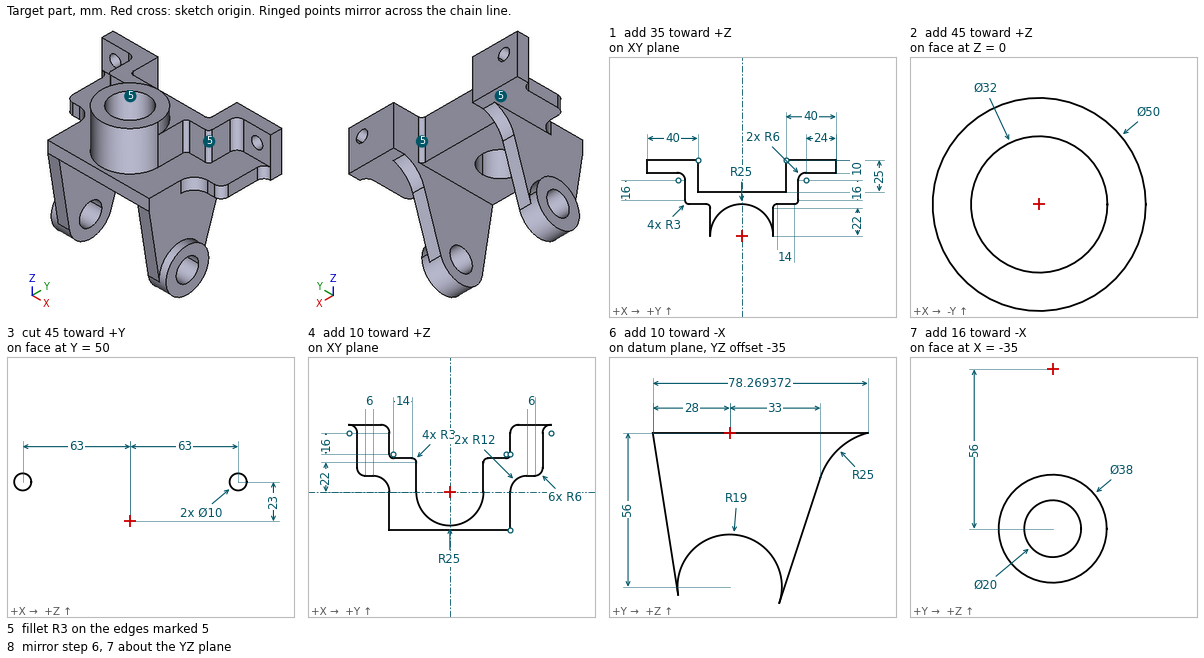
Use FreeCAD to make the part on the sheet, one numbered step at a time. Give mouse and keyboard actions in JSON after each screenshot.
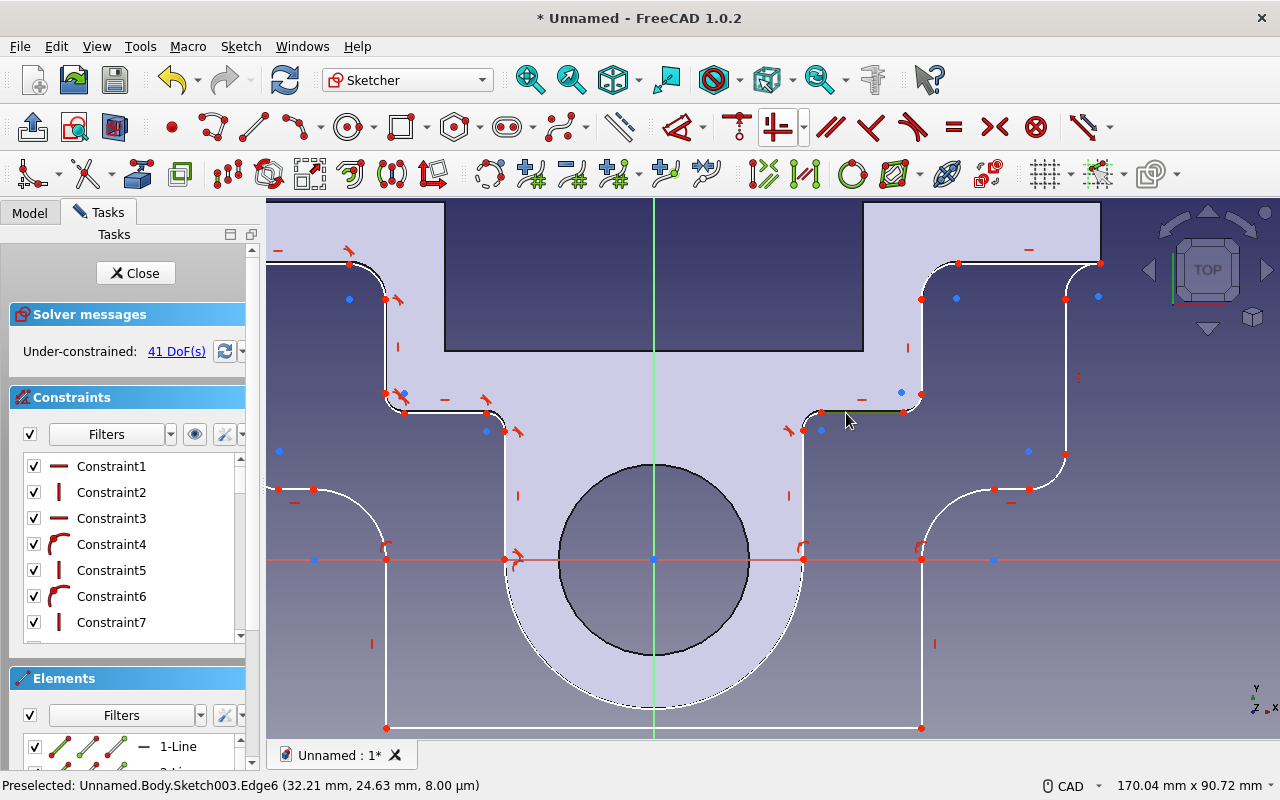
{"action": "left_click", "coordinate": [809, 418]}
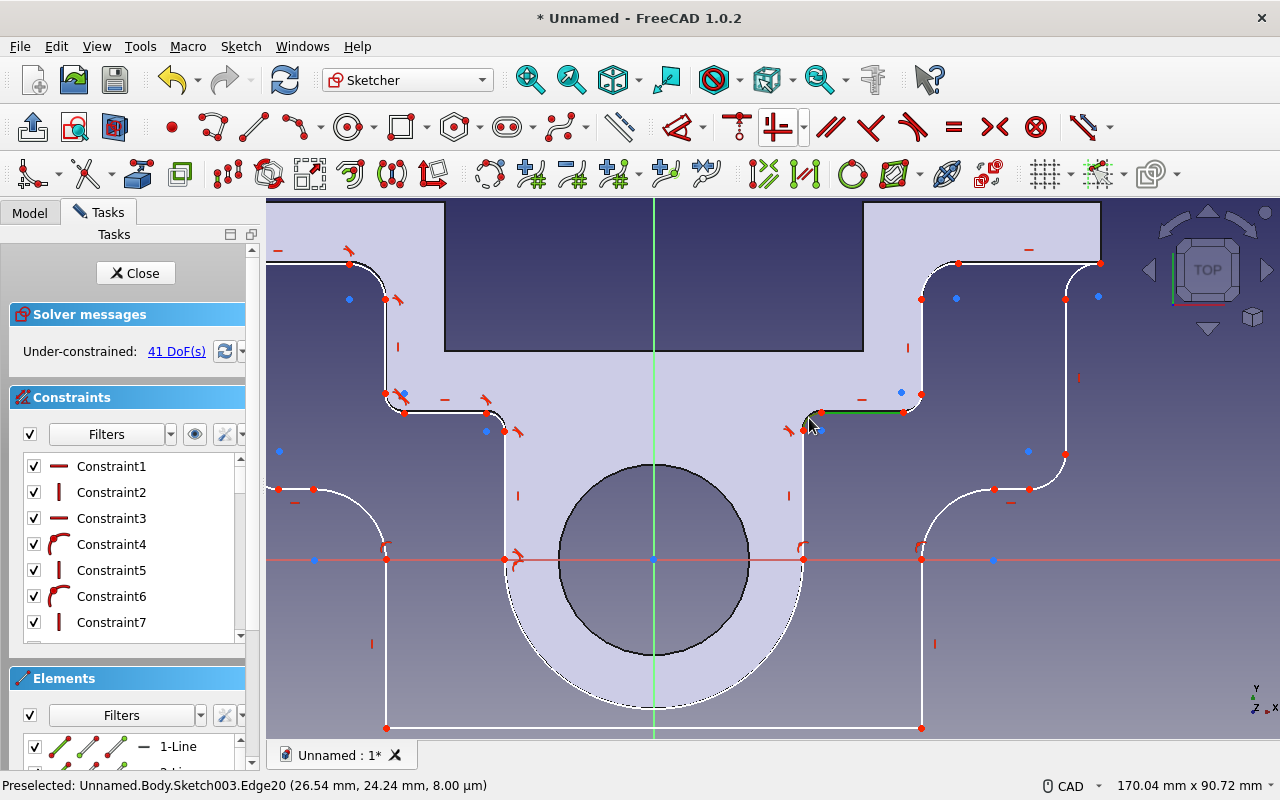
{"action": "left_click", "coordinate": [913, 128]}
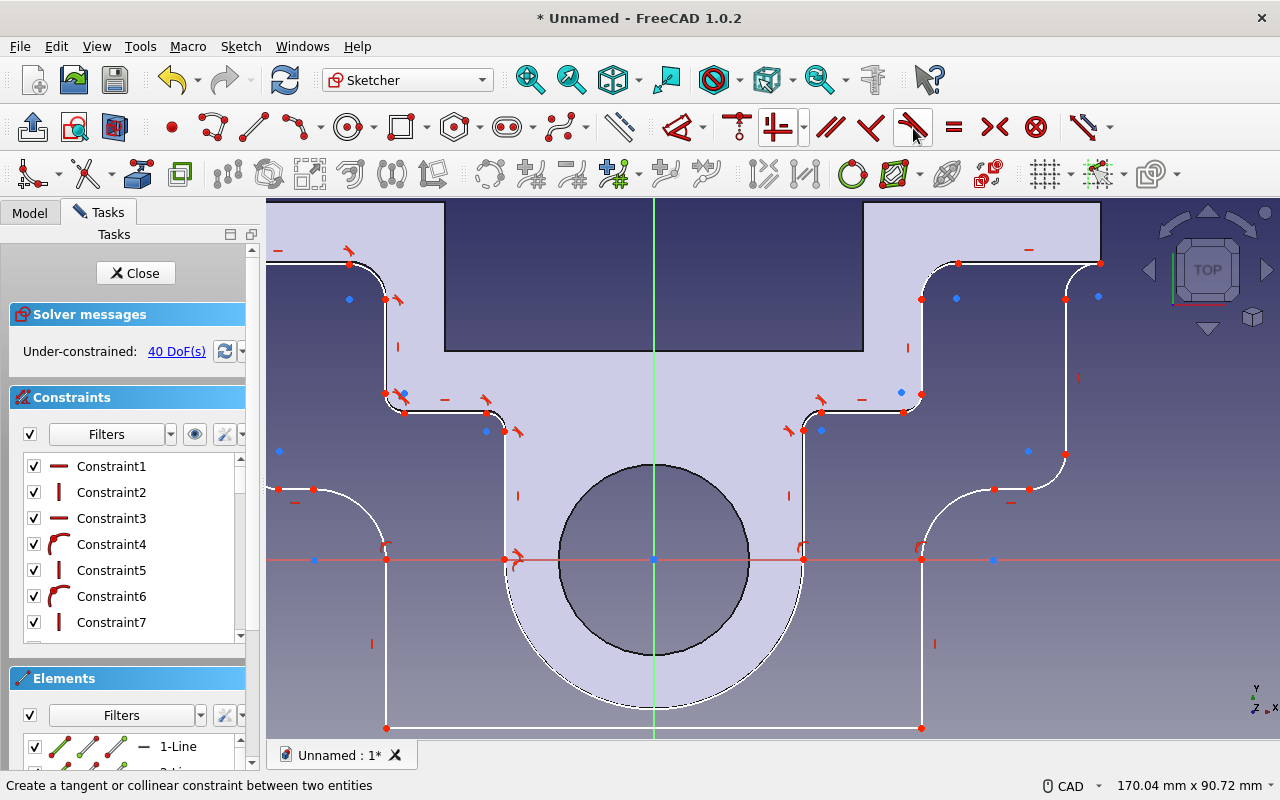
{"action": "left_click", "coordinate": [846, 413]}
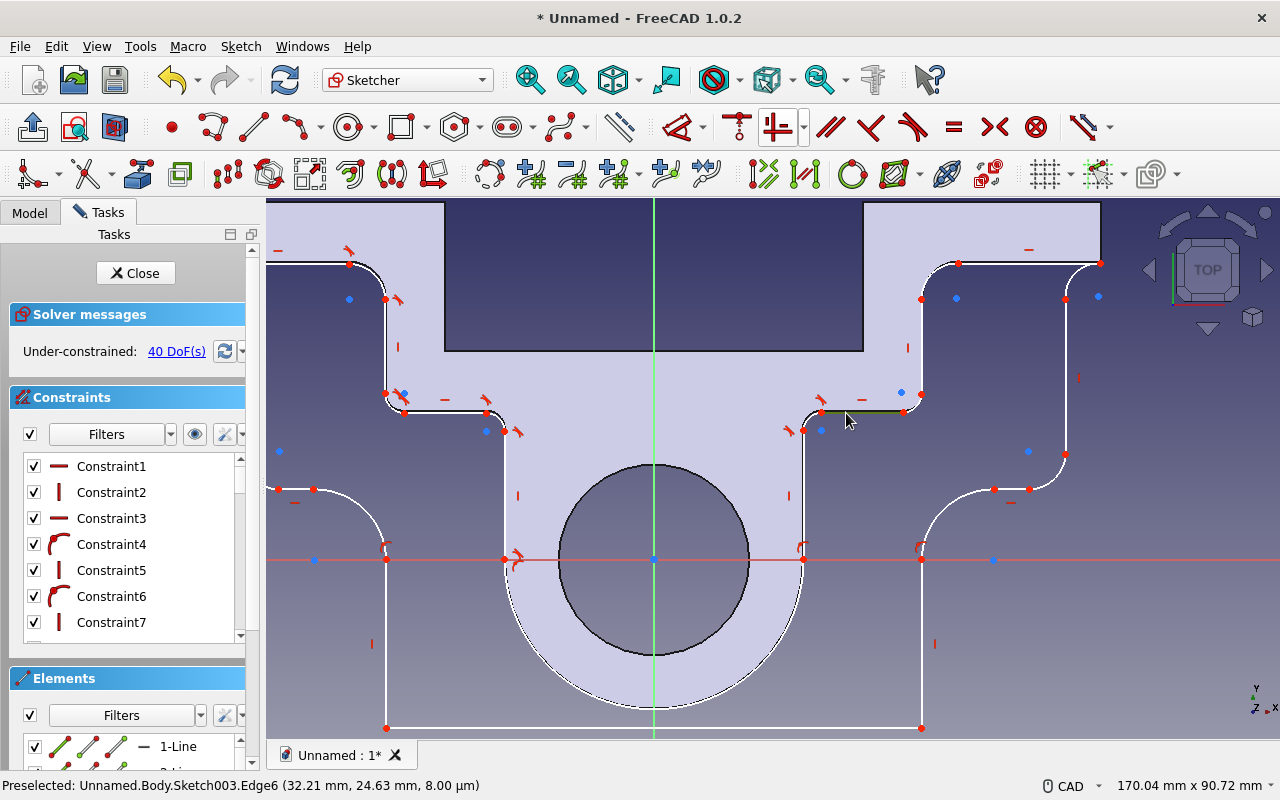
{"action": "left_click", "coordinate": [916, 407]}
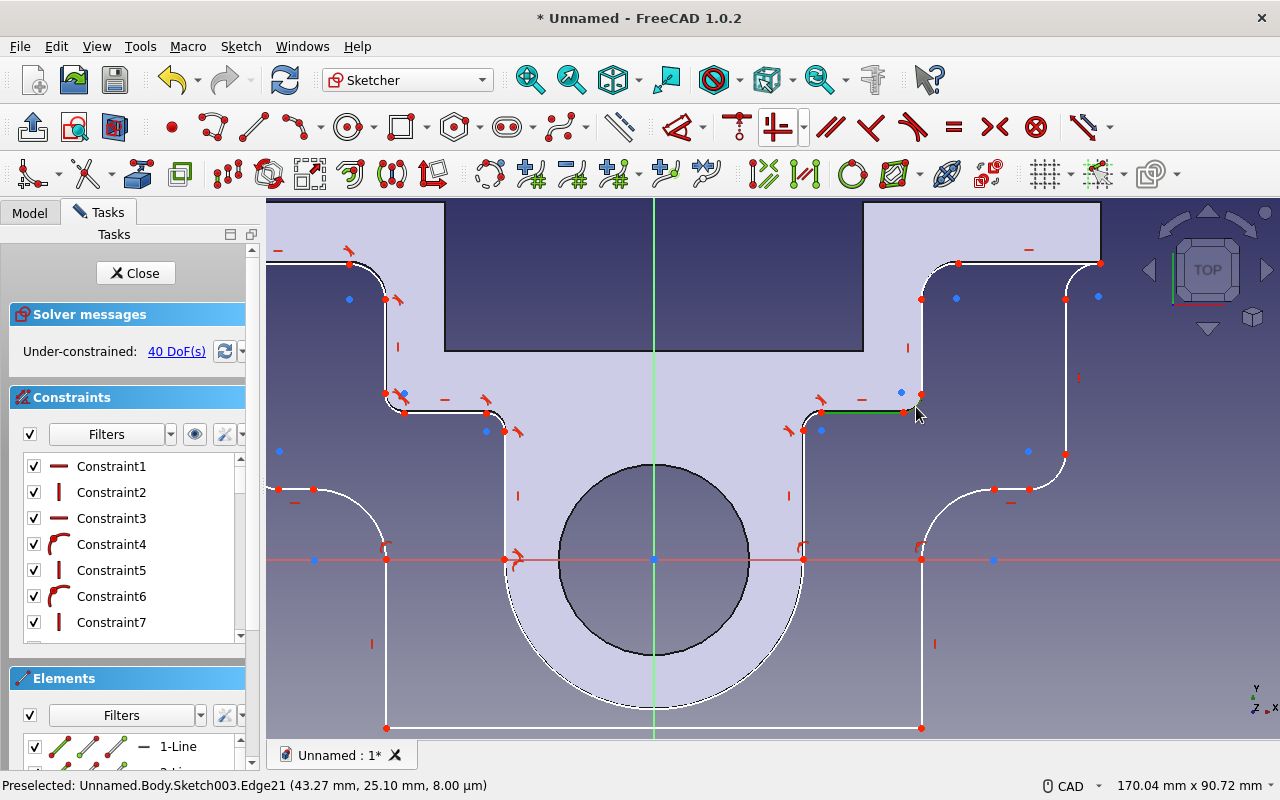
{"action": "left_click", "coordinate": [913, 128]}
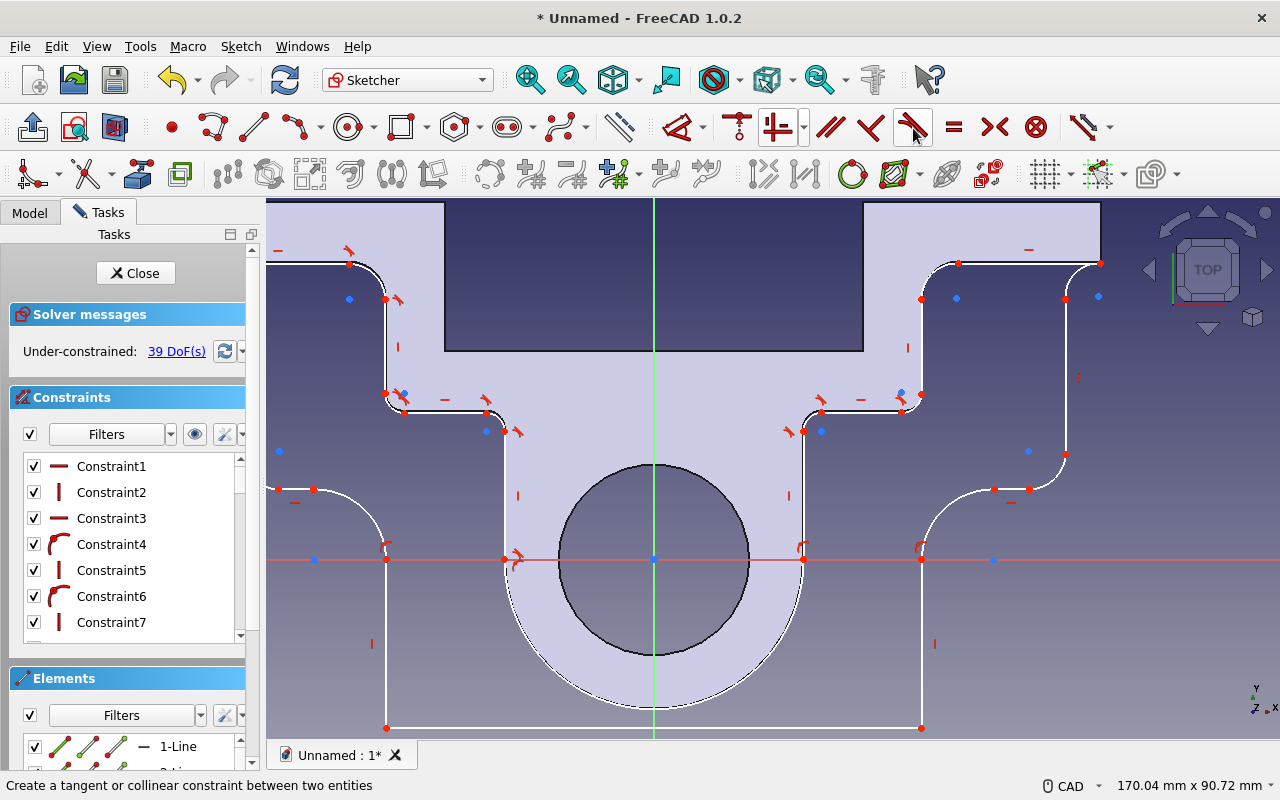
{"action": "left_click", "coordinate": [922, 366]}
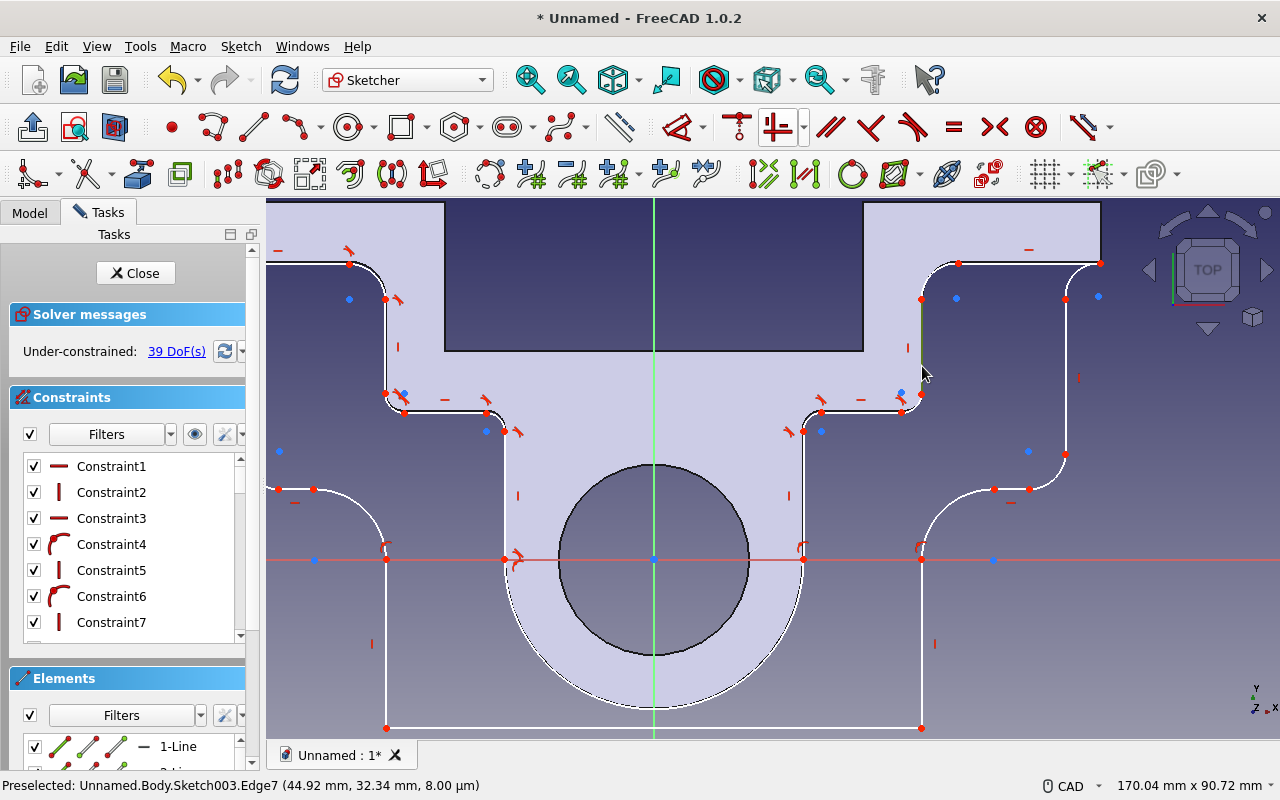
{"action": "left_click", "coordinate": [915, 408]}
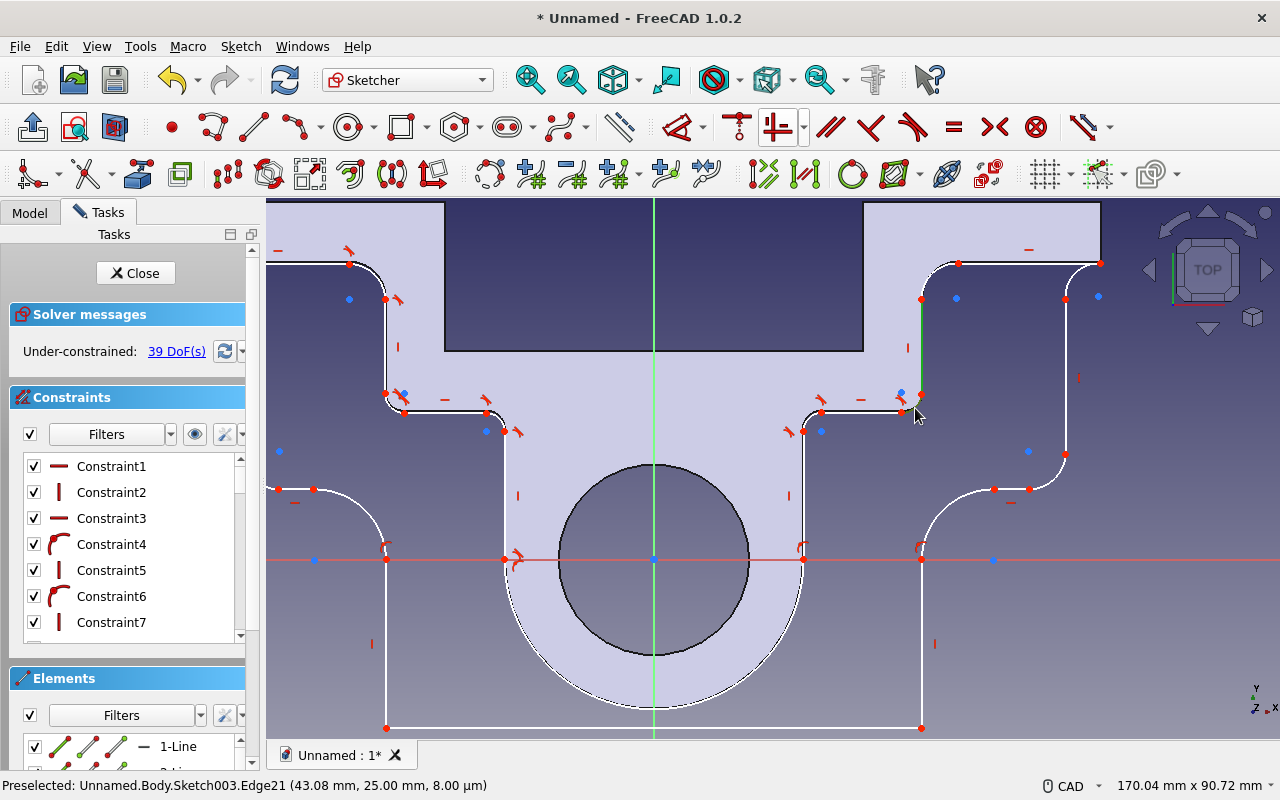
{"action": "left_click", "coordinate": [913, 128]}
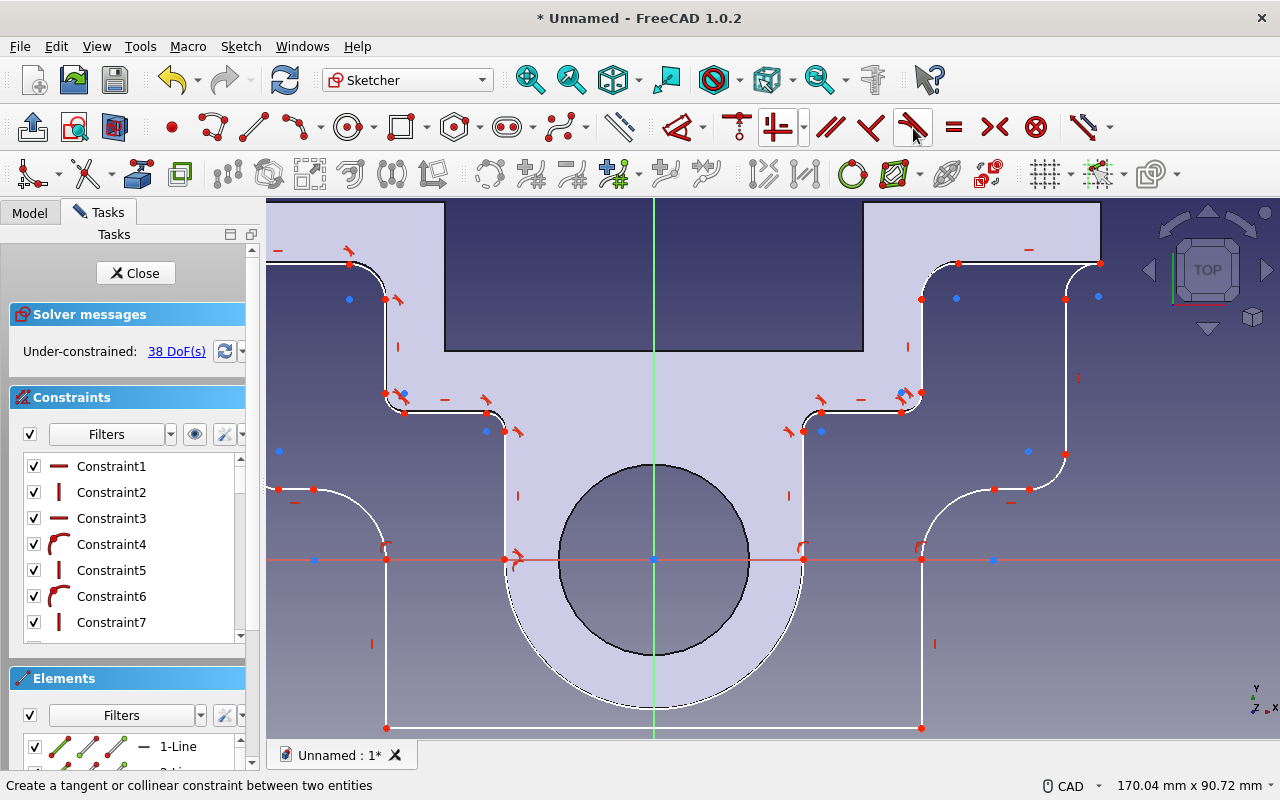
{"action": "left_click", "coordinate": [922, 365]}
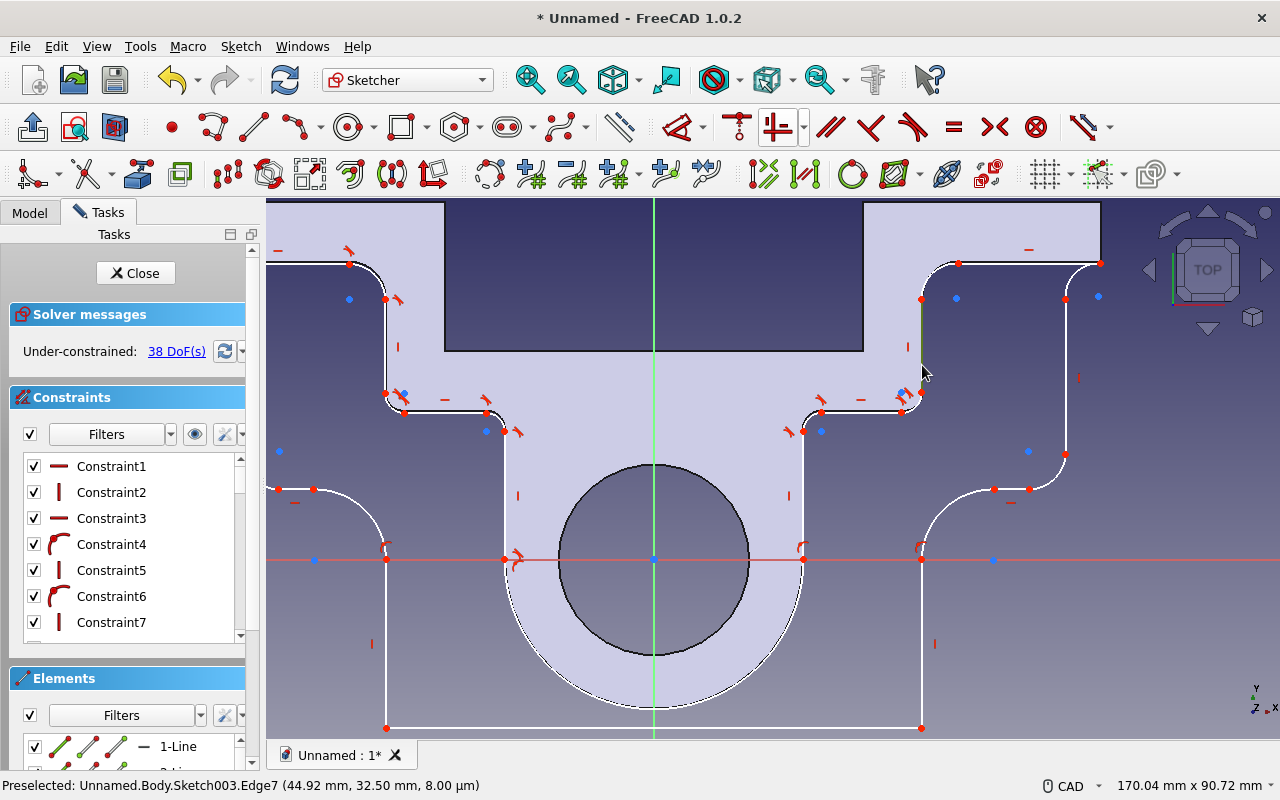
{"action": "left_click", "coordinate": [941, 267]}